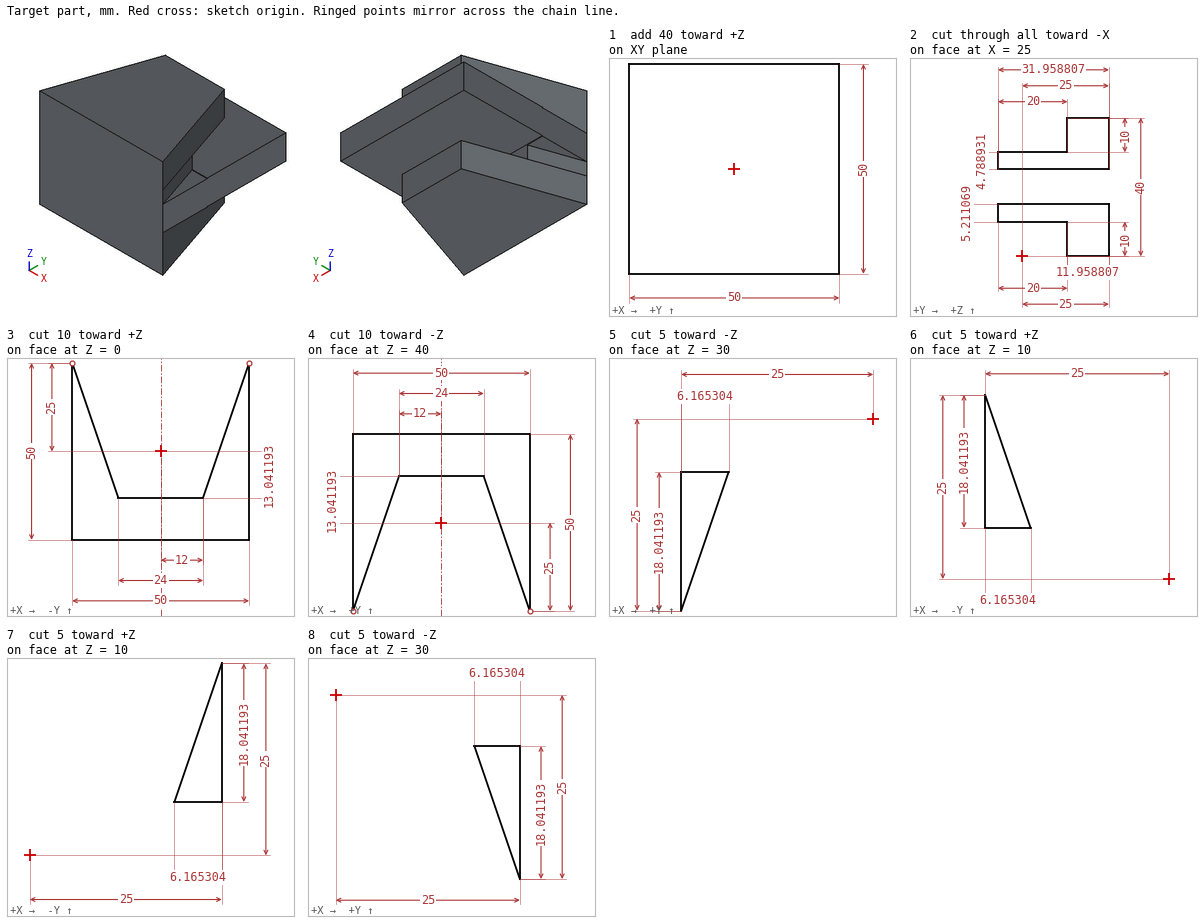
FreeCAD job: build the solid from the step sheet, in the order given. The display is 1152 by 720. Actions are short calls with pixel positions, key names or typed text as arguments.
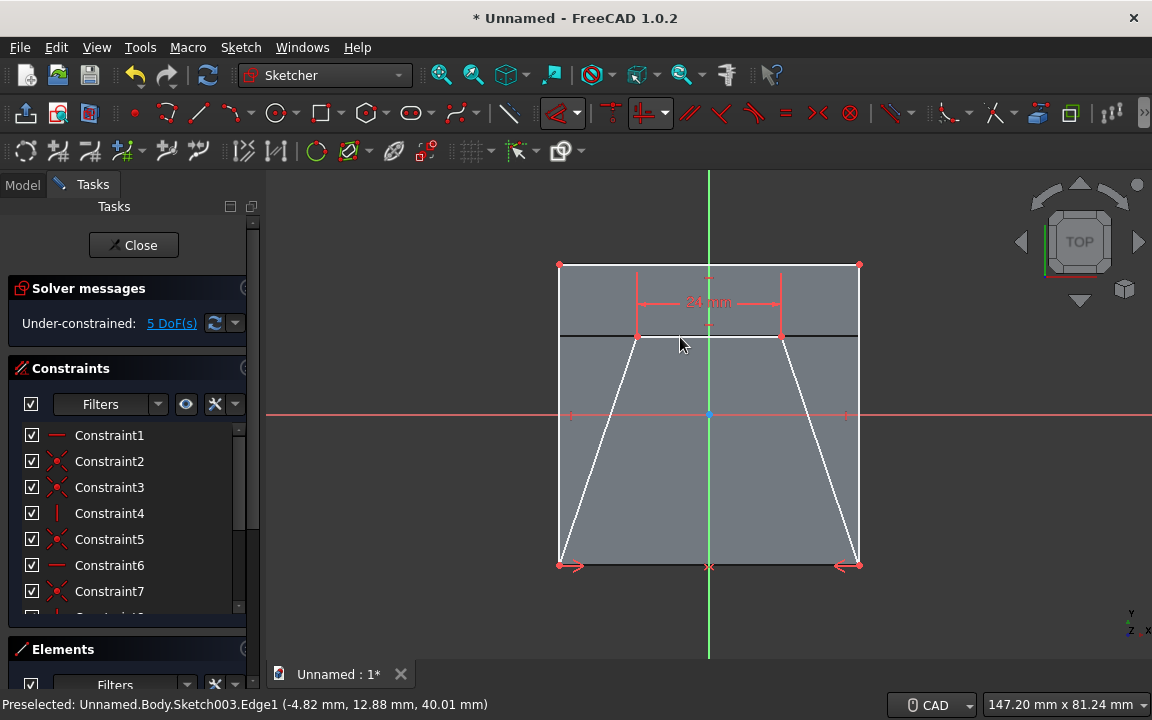
click(859, 476)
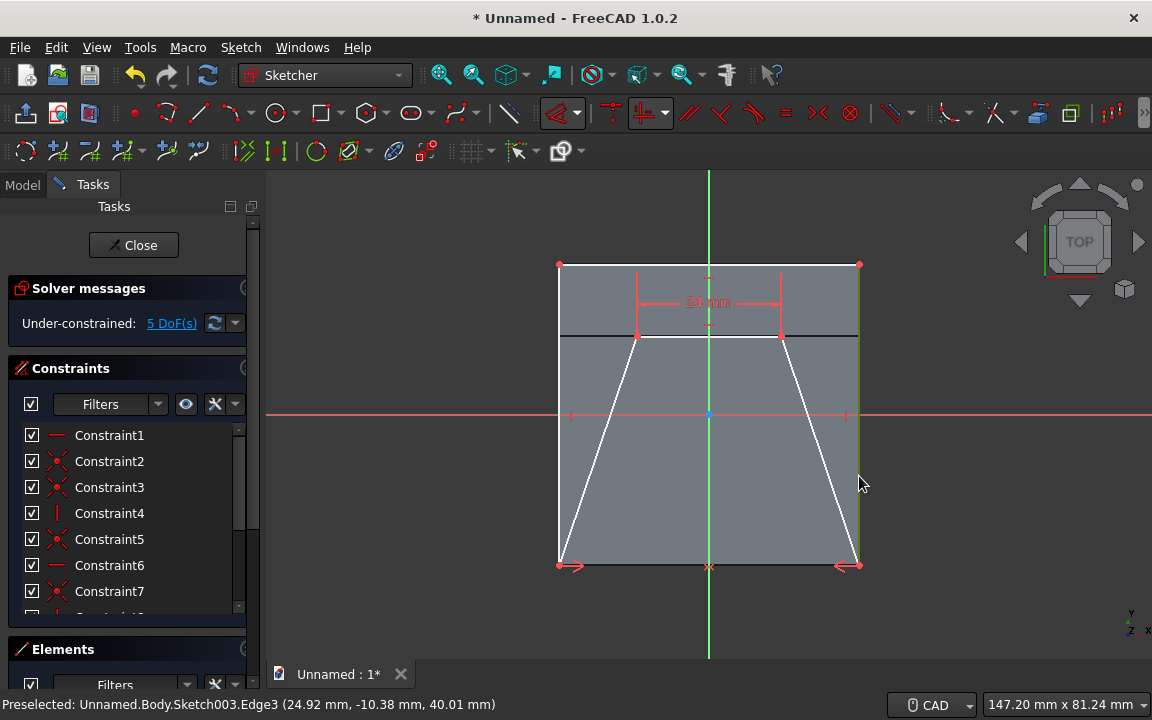
key(i)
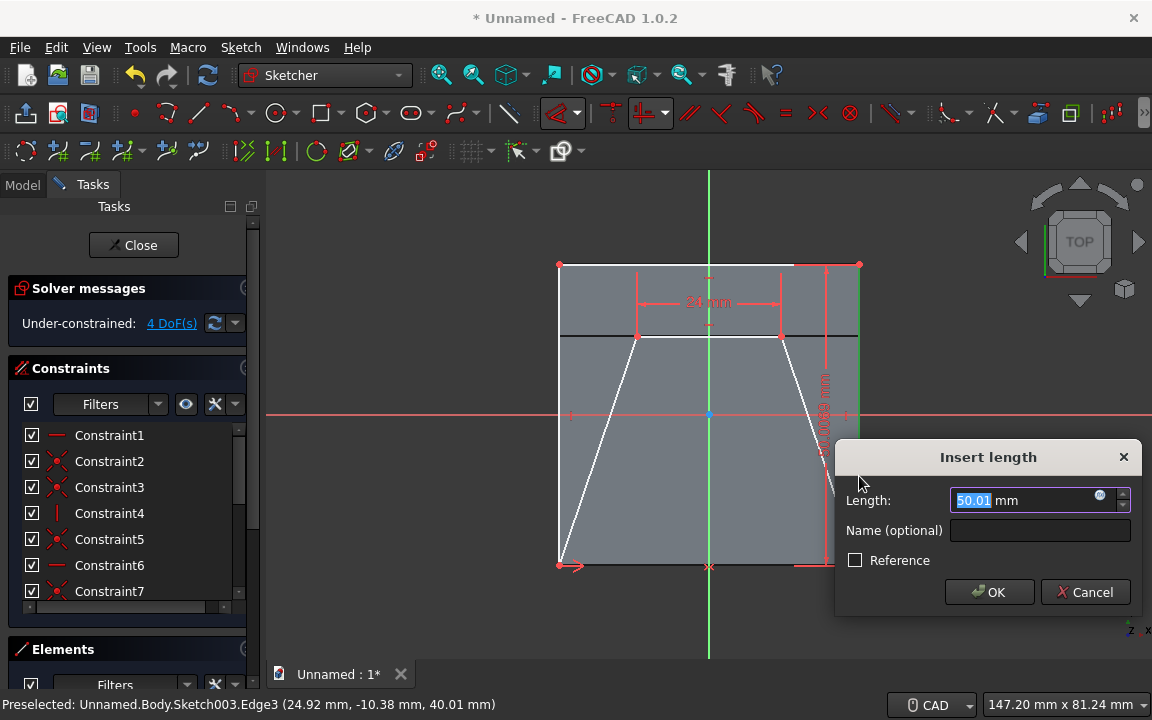
text(50)
key(Return)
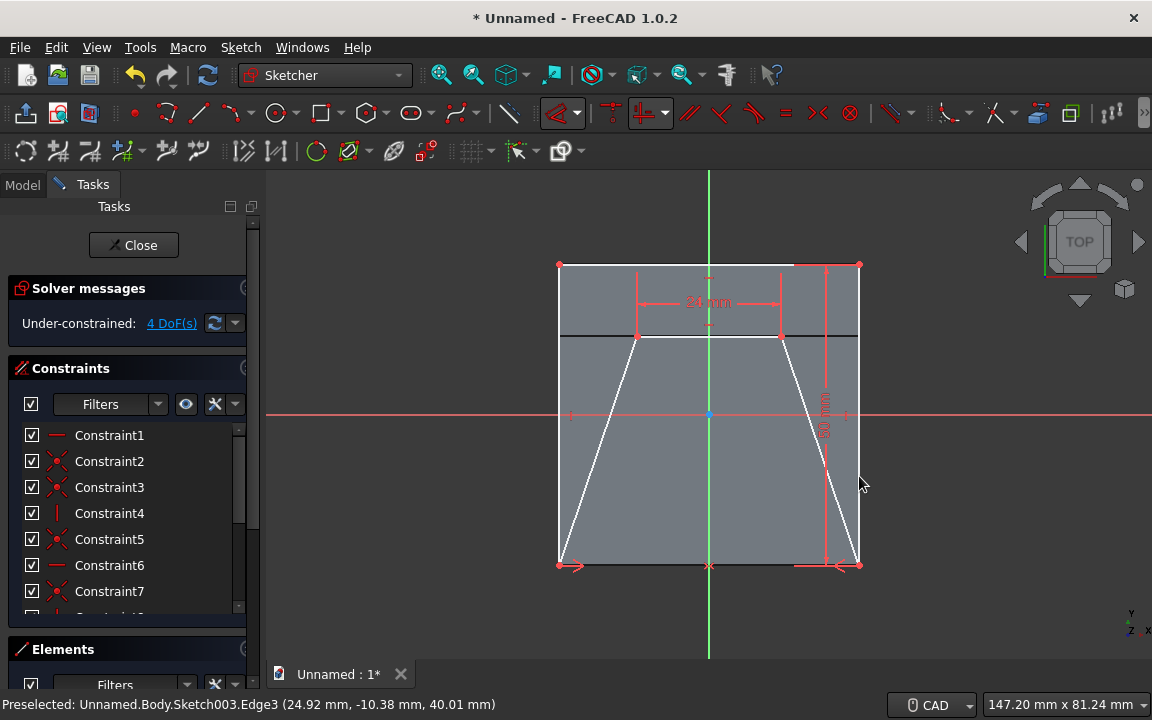
click(769, 265)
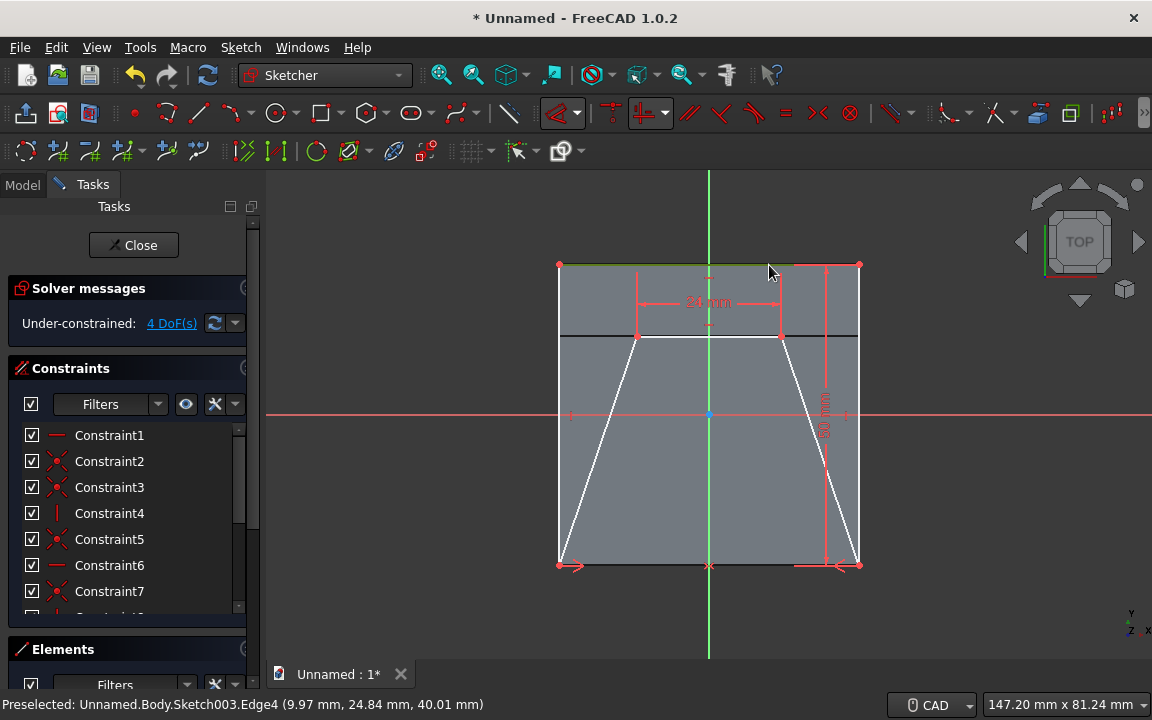
key(l)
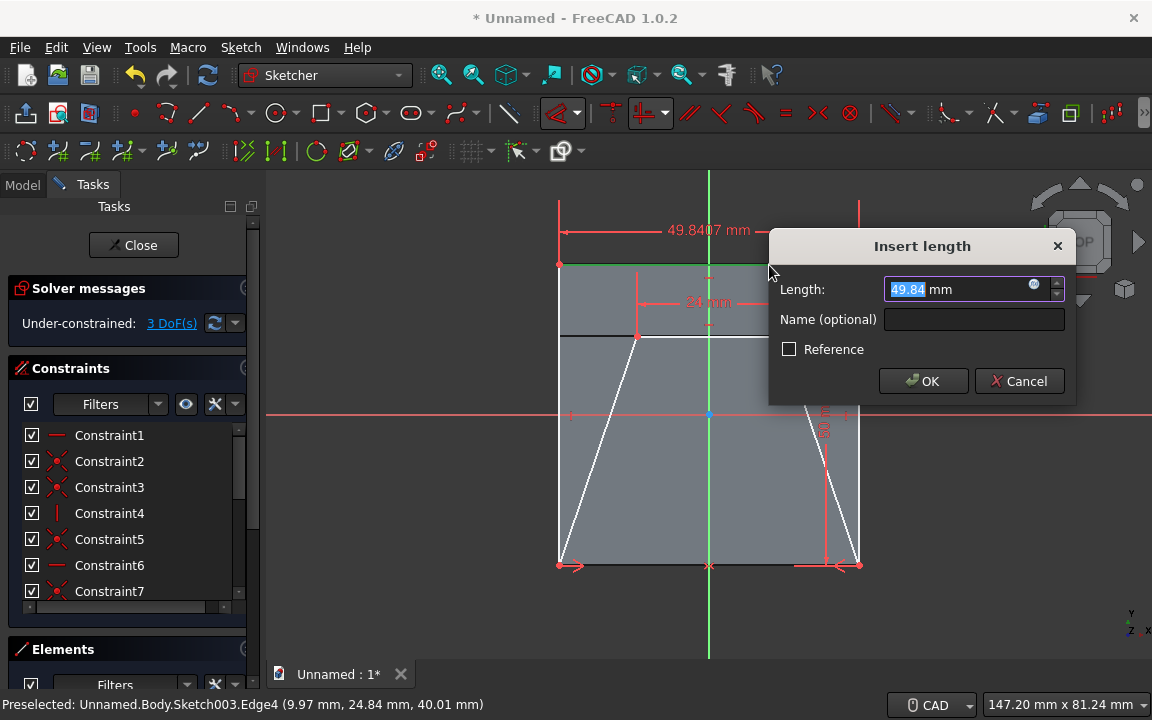
text(50)
key(Return)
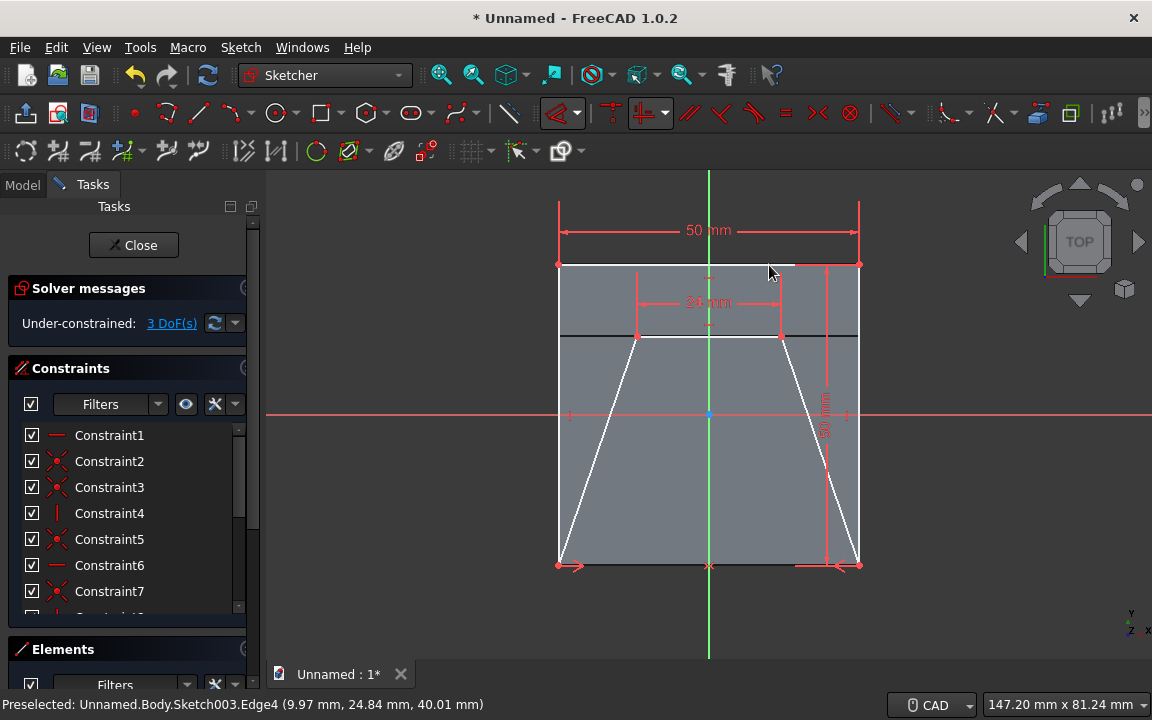
click(637, 337)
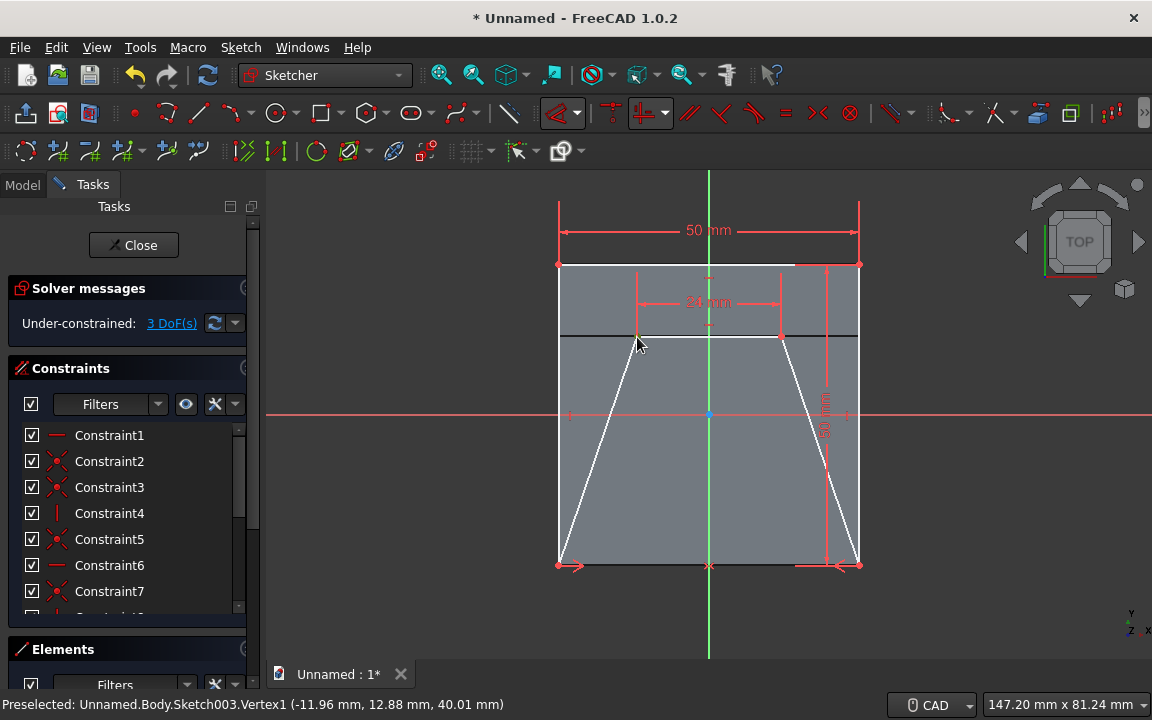
click(580, 114)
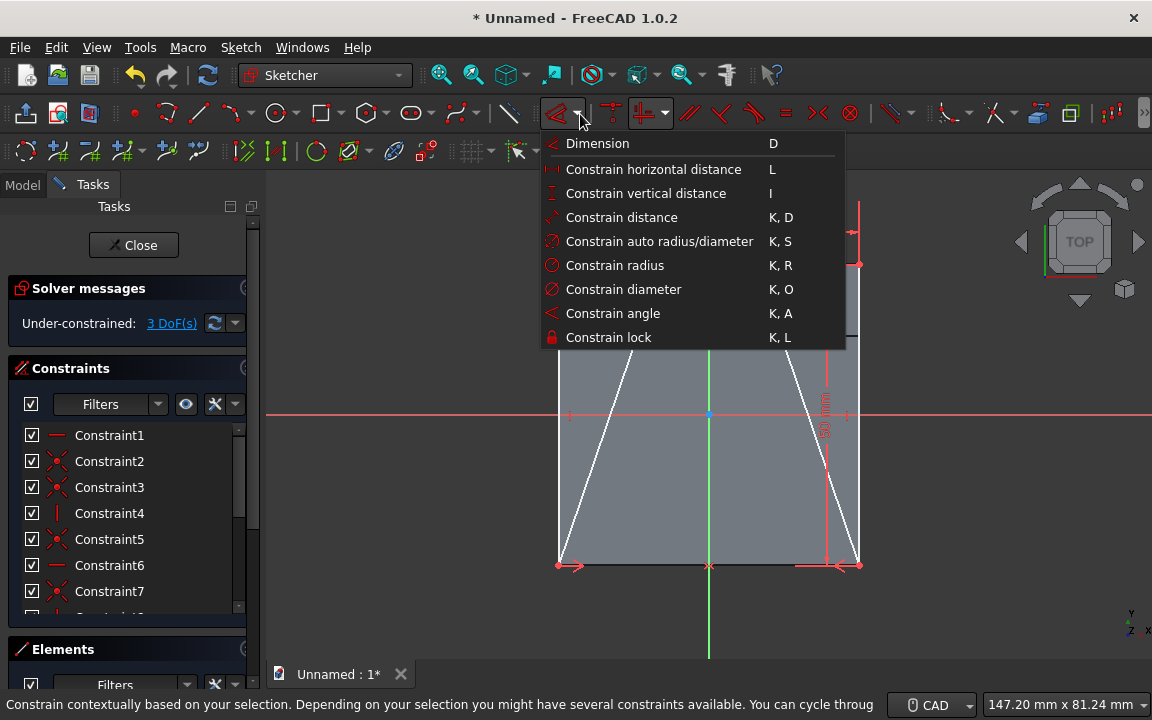
click(693, 169)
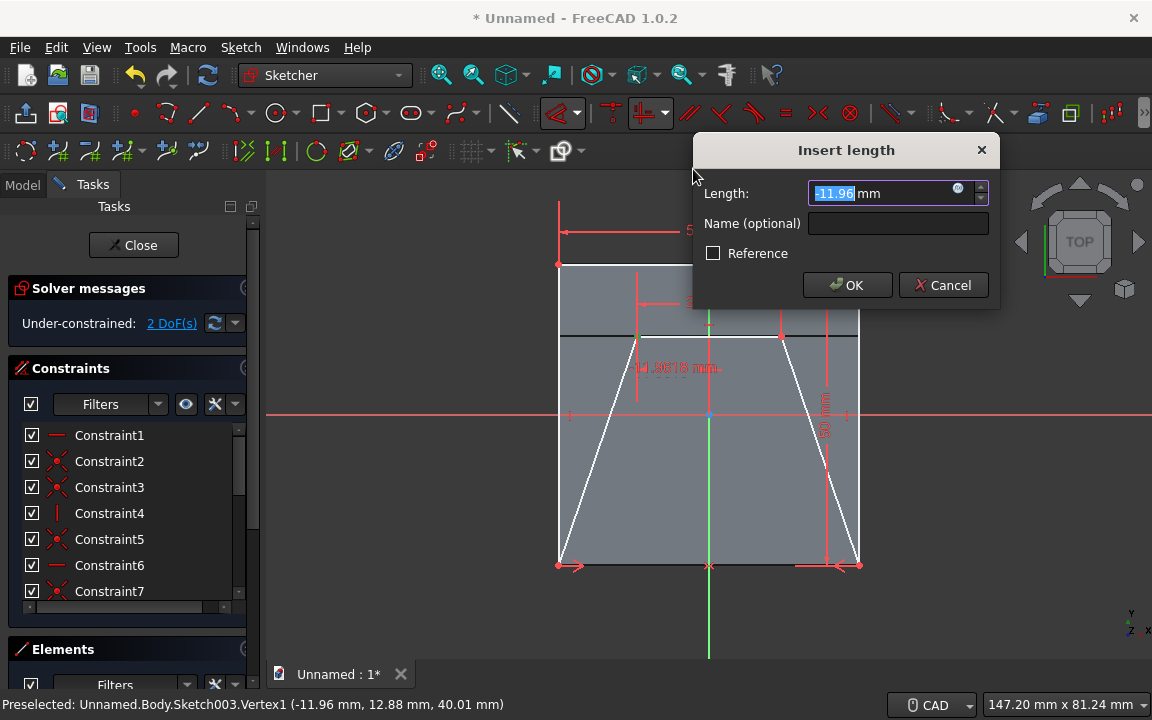
text(-12)
key(Return)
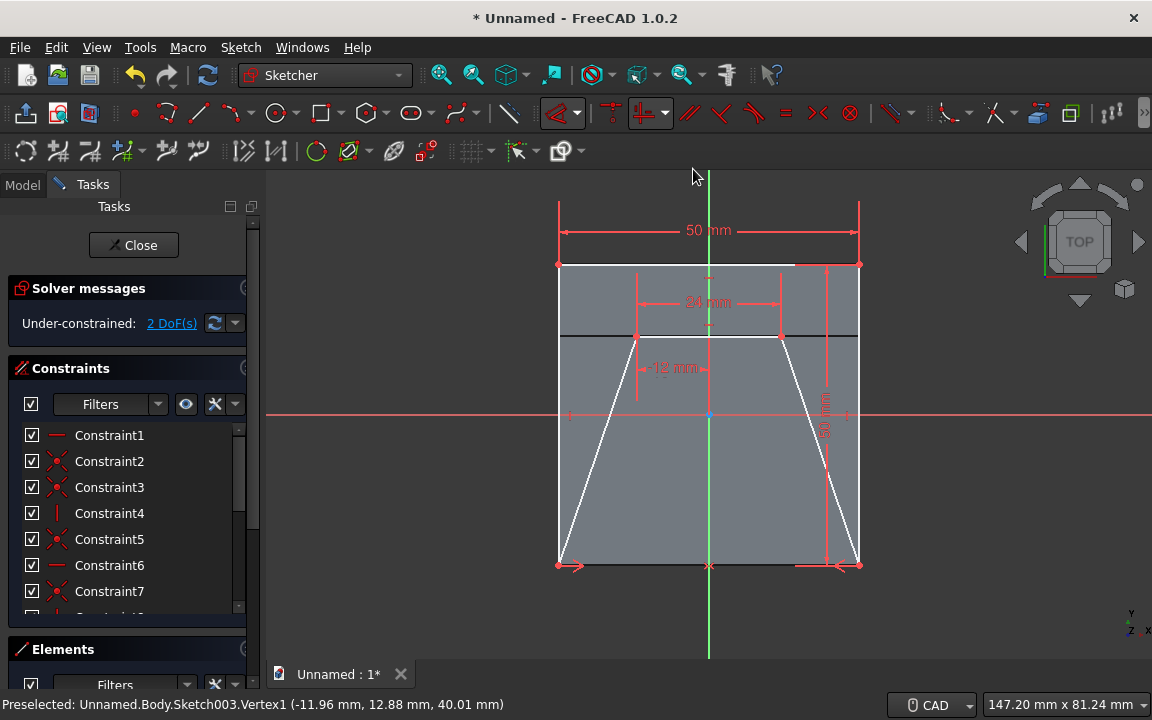
click(859, 566)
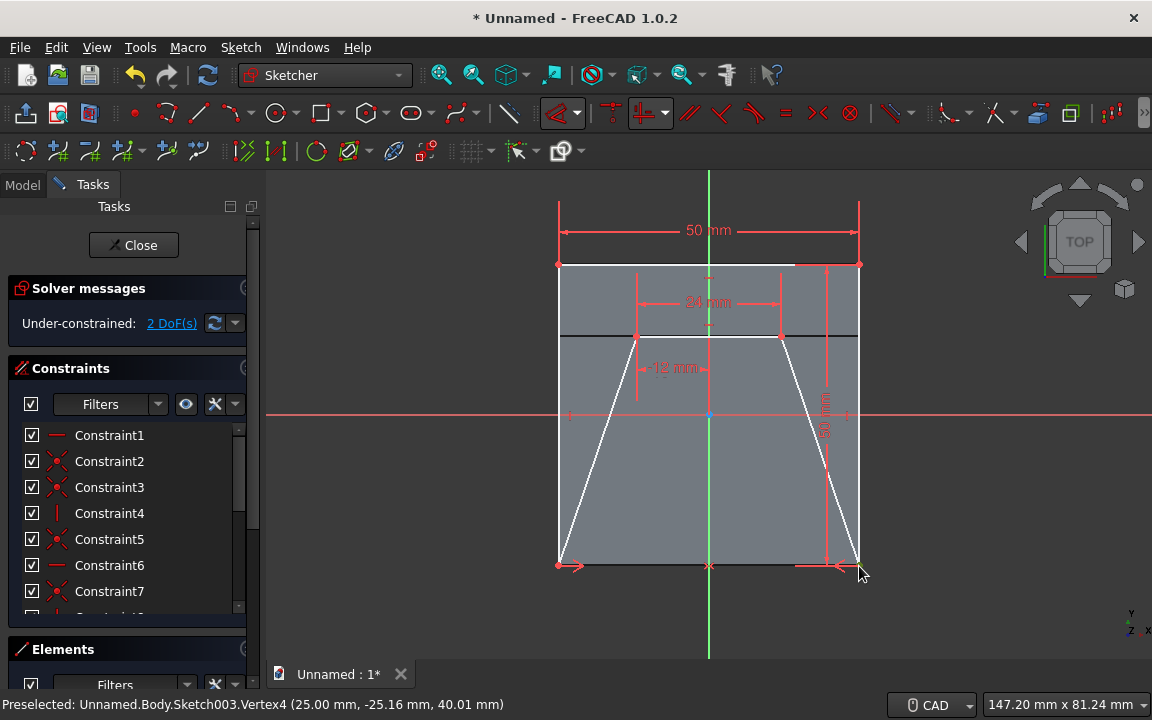
key(i)